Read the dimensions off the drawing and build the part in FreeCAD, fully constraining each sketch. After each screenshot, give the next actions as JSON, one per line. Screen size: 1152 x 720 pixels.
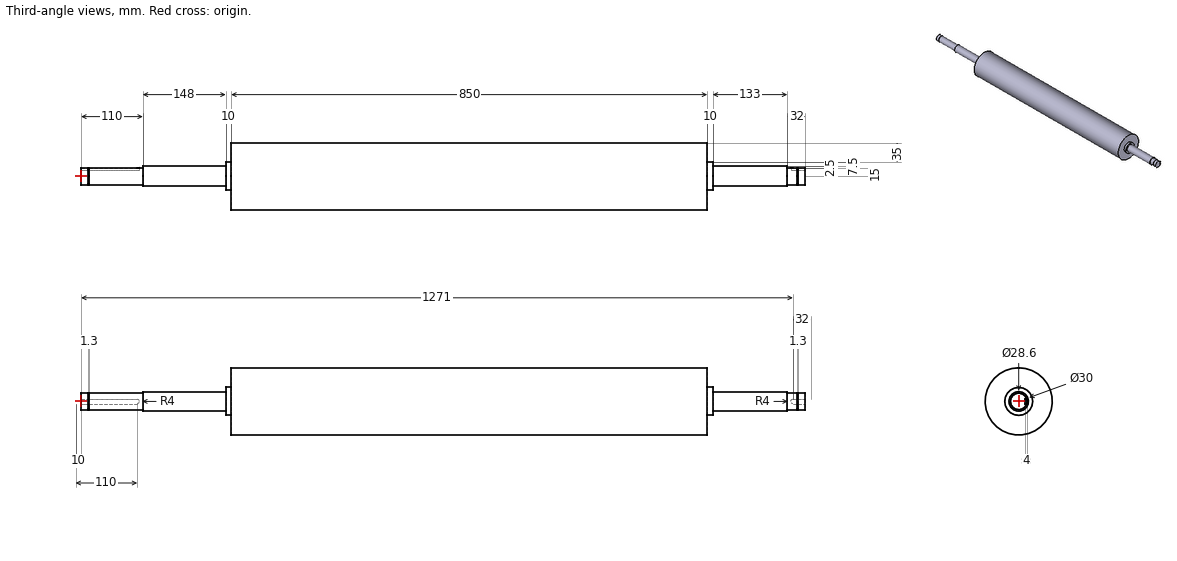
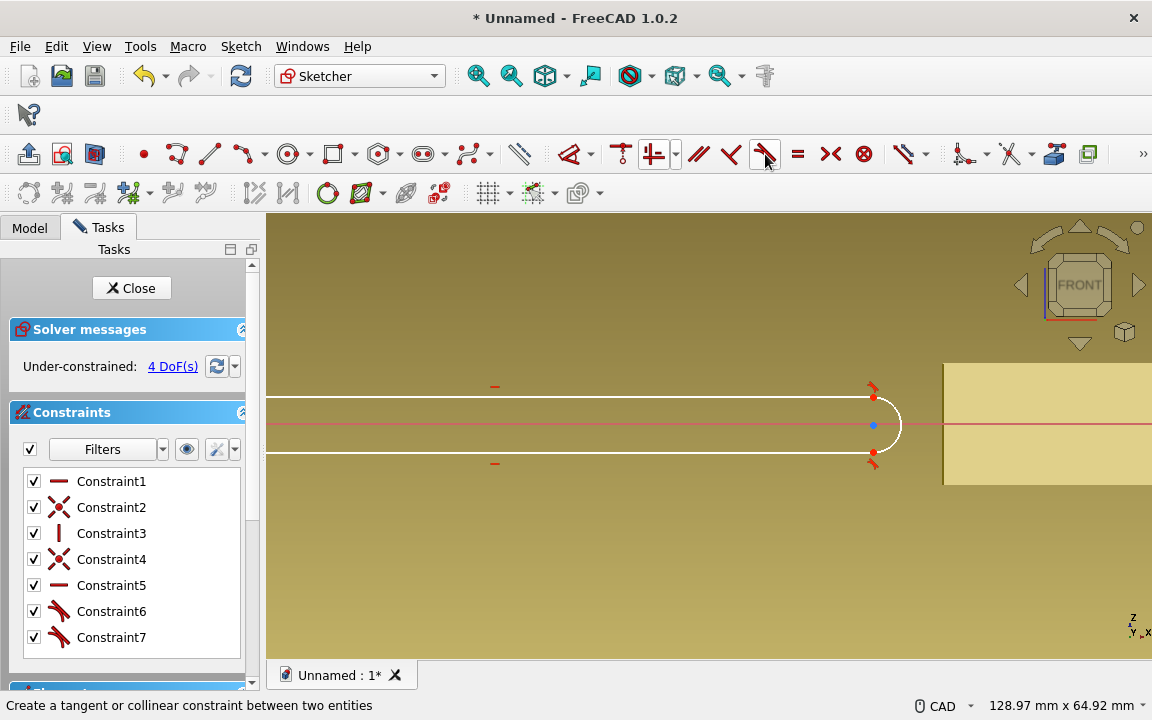
{"action": "left_click", "coordinate": [873, 425]}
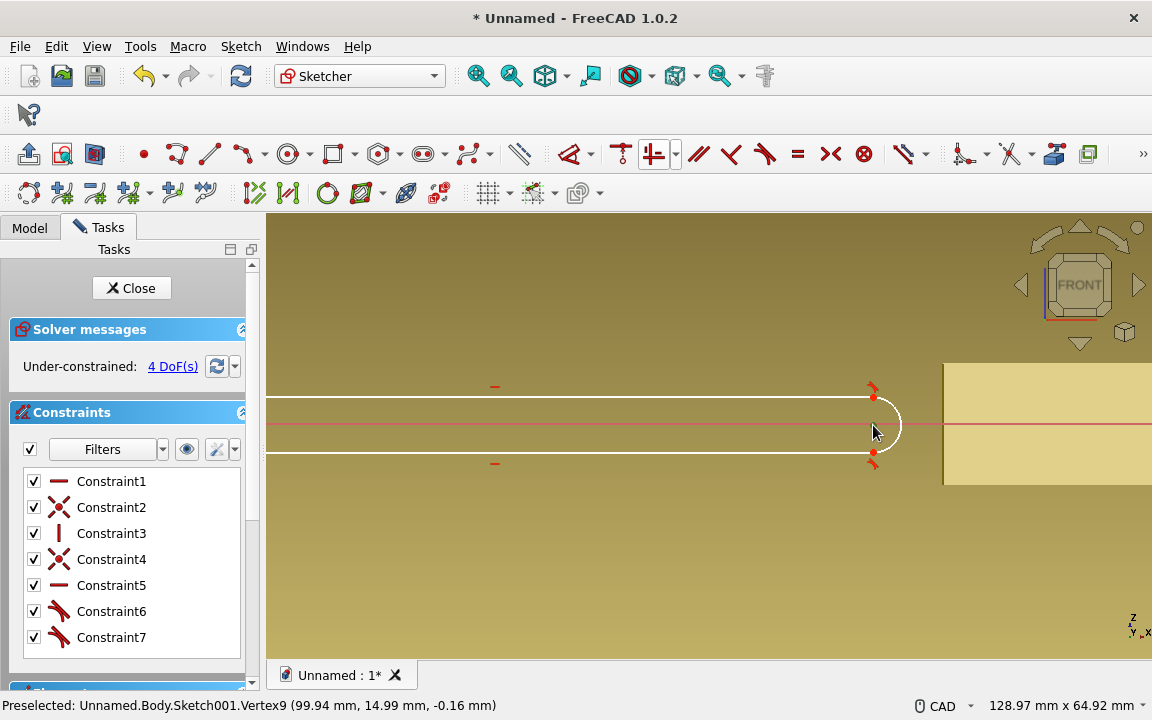
{"action": "left_click", "coordinate": [938, 424]}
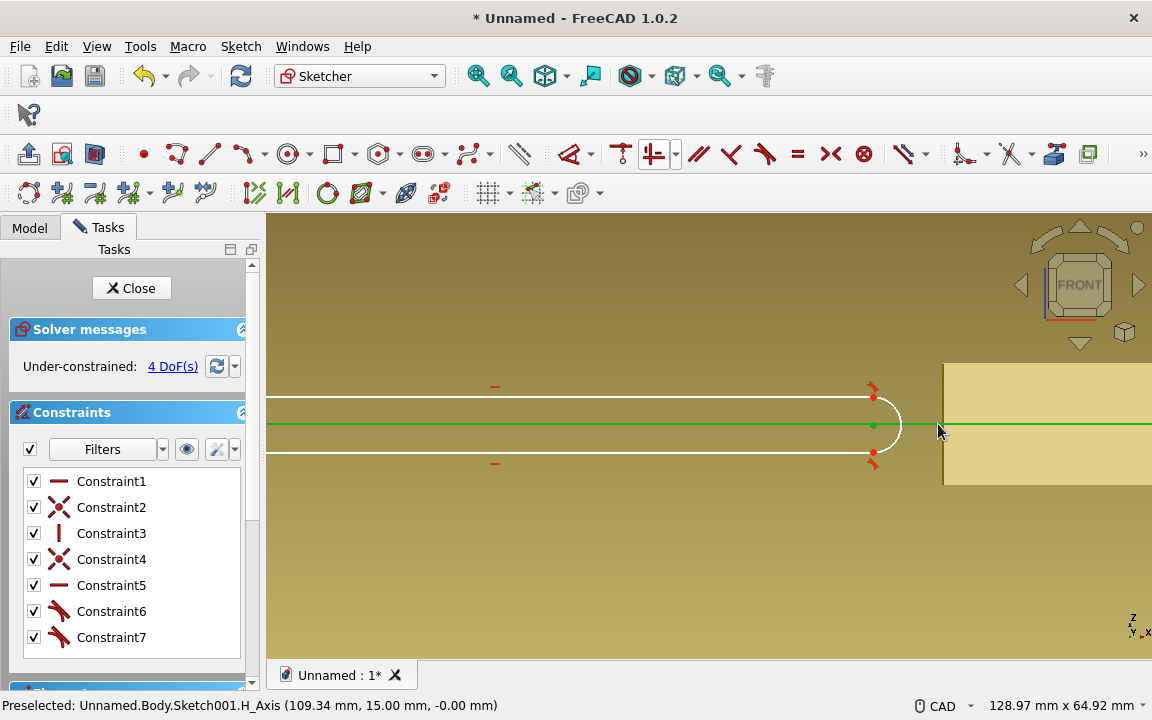
{"action": "left_click", "coordinate": [621, 154]}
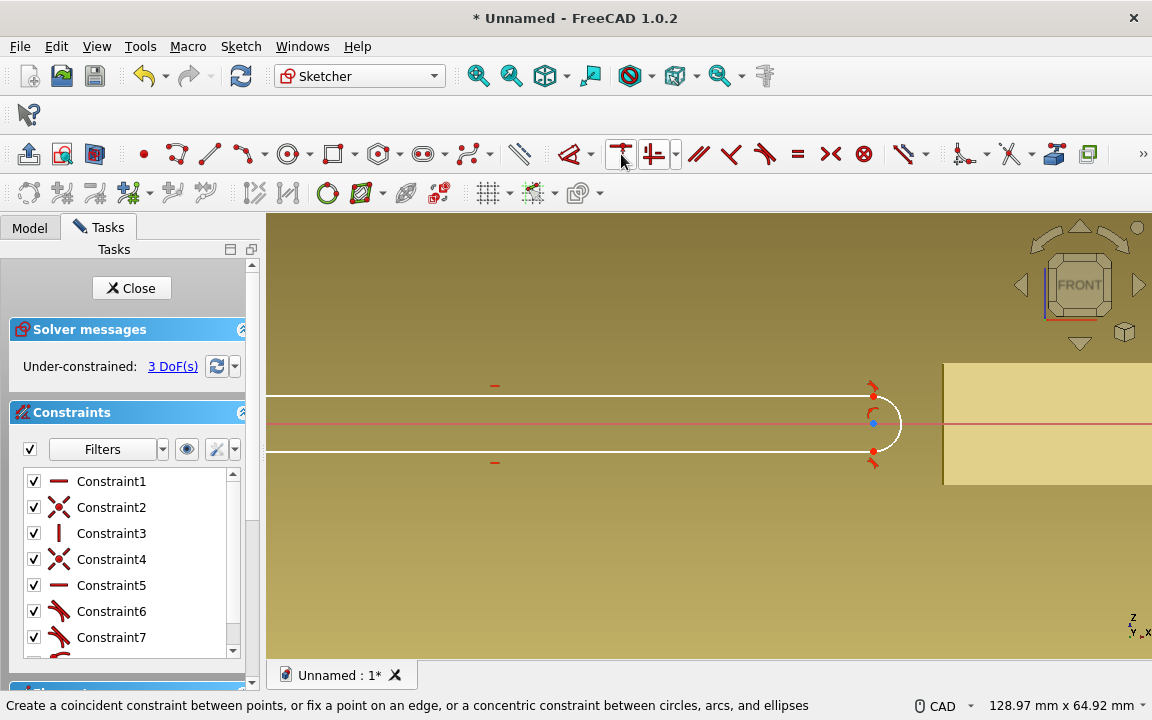
{"action": "key", "text": "d"}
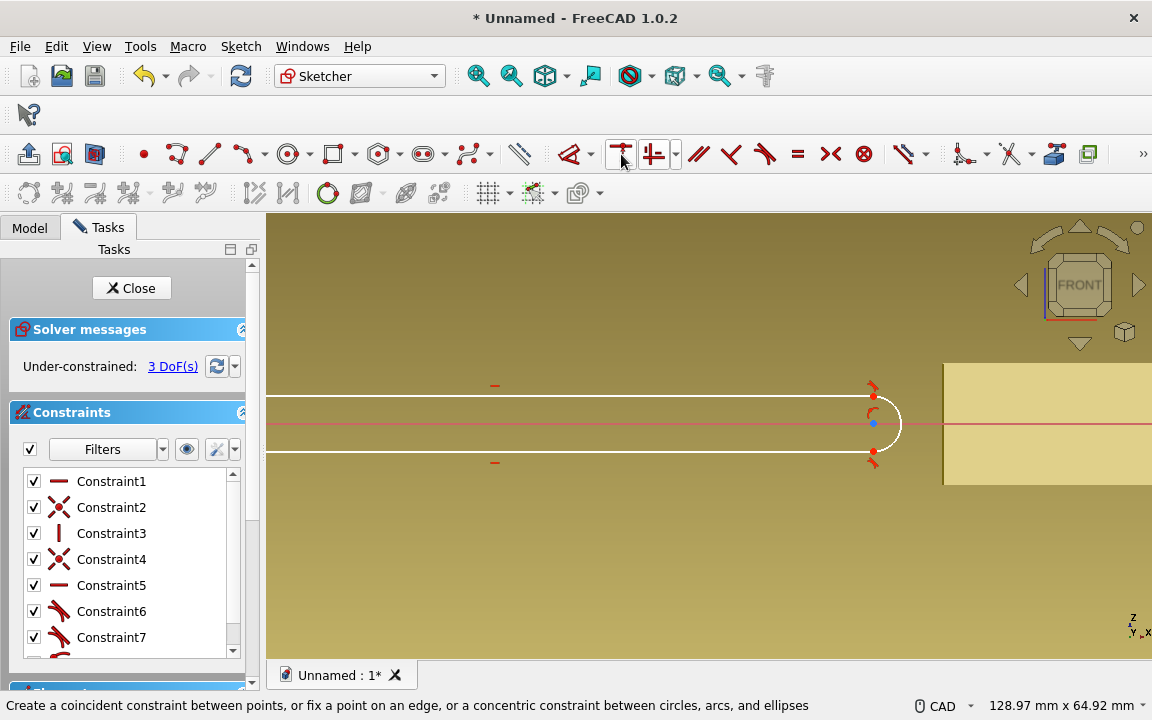
{"action": "scroll", "coordinate": [896, 440], "scroll_direction": "up", "scroll_amount": 2}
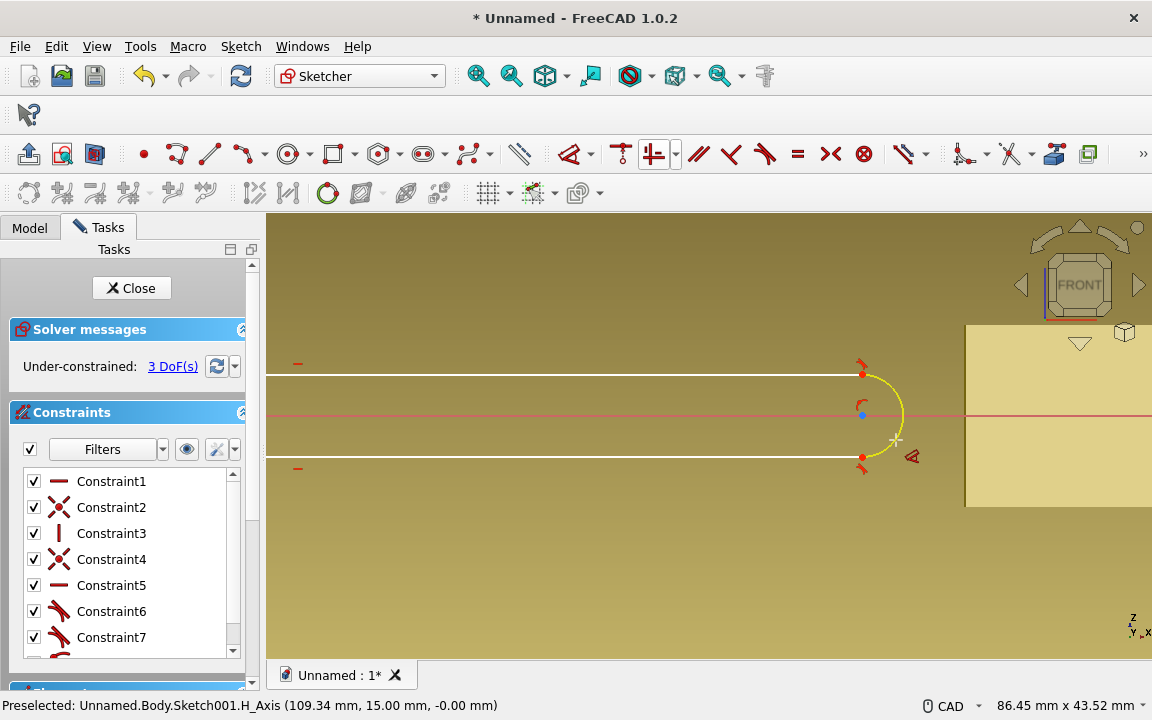
{"action": "left_click", "coordinate": [895, 440]}
{"action": "left_click", "coordinate": [921, 459]}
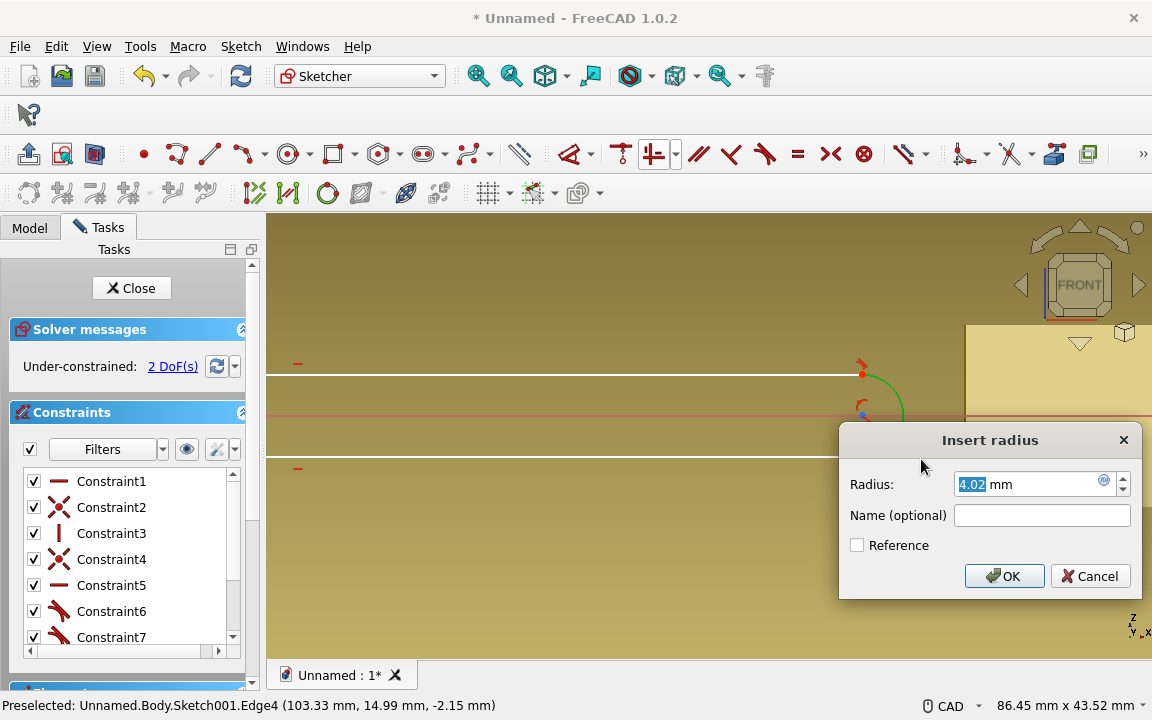
{"action": "type", "text": "4"}
{"action": "key", "text": "Return"}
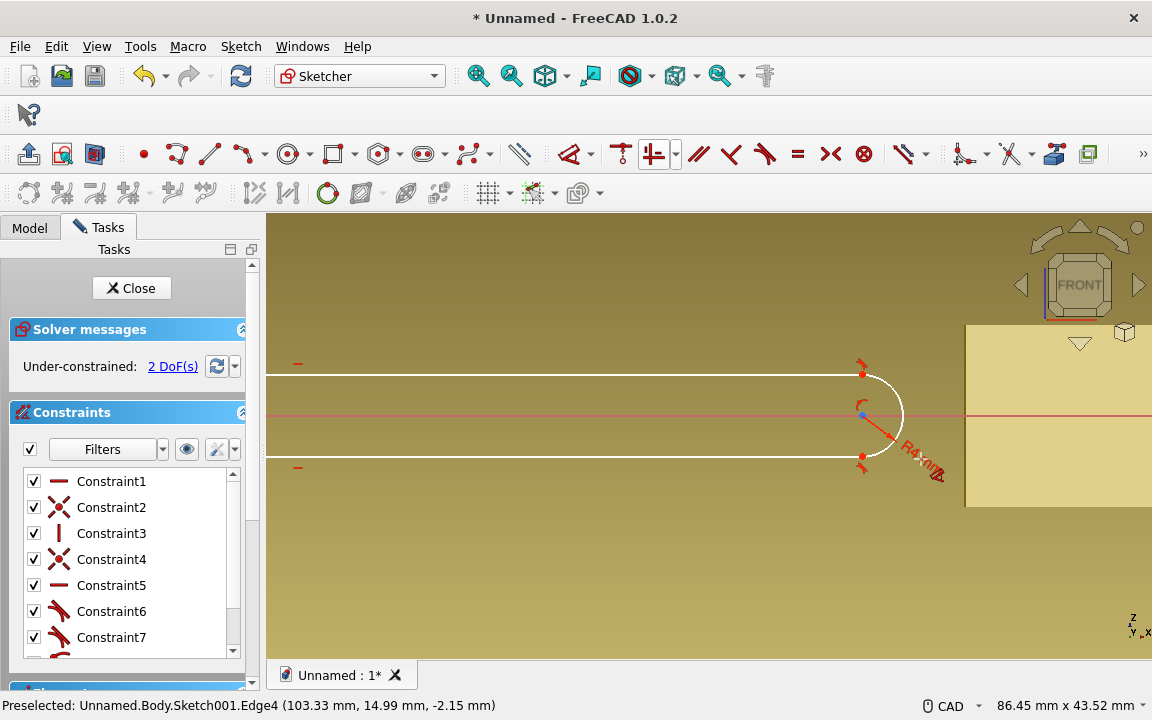
{"action": "left_click", "coordinate": [524, 457]}
{"action": "left_click", "coordinate": [578, 491]}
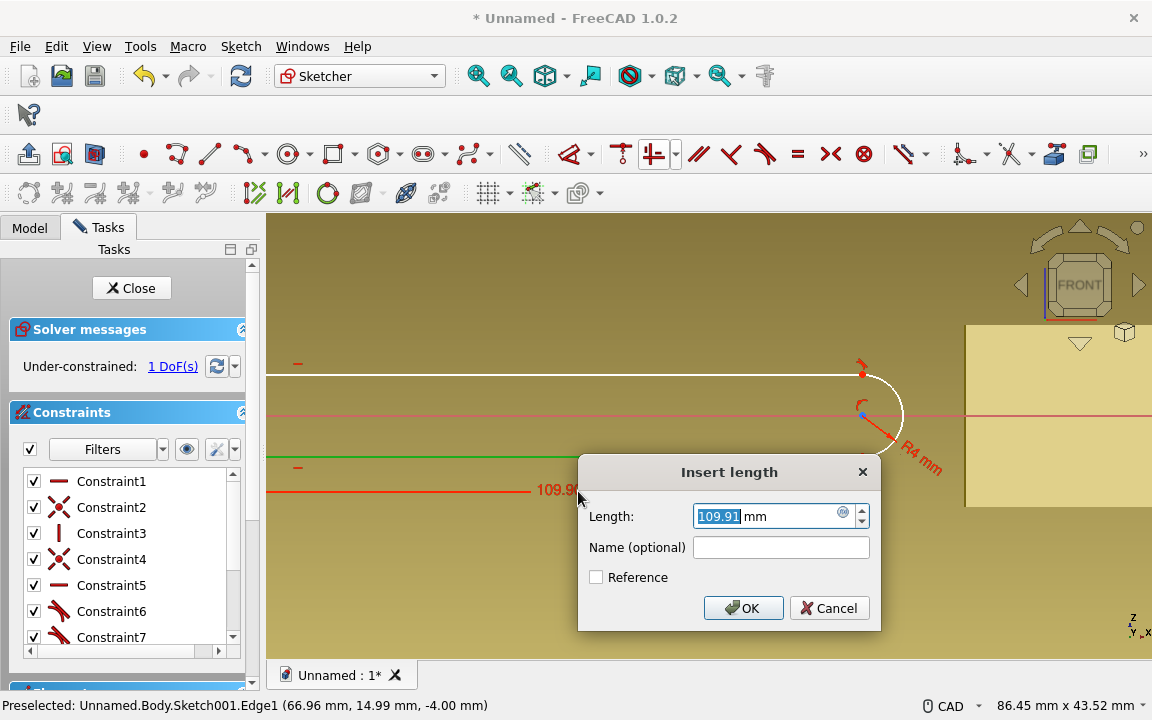
{"action": "type", "text": "110"}
{"action": "key", "text": "Return"}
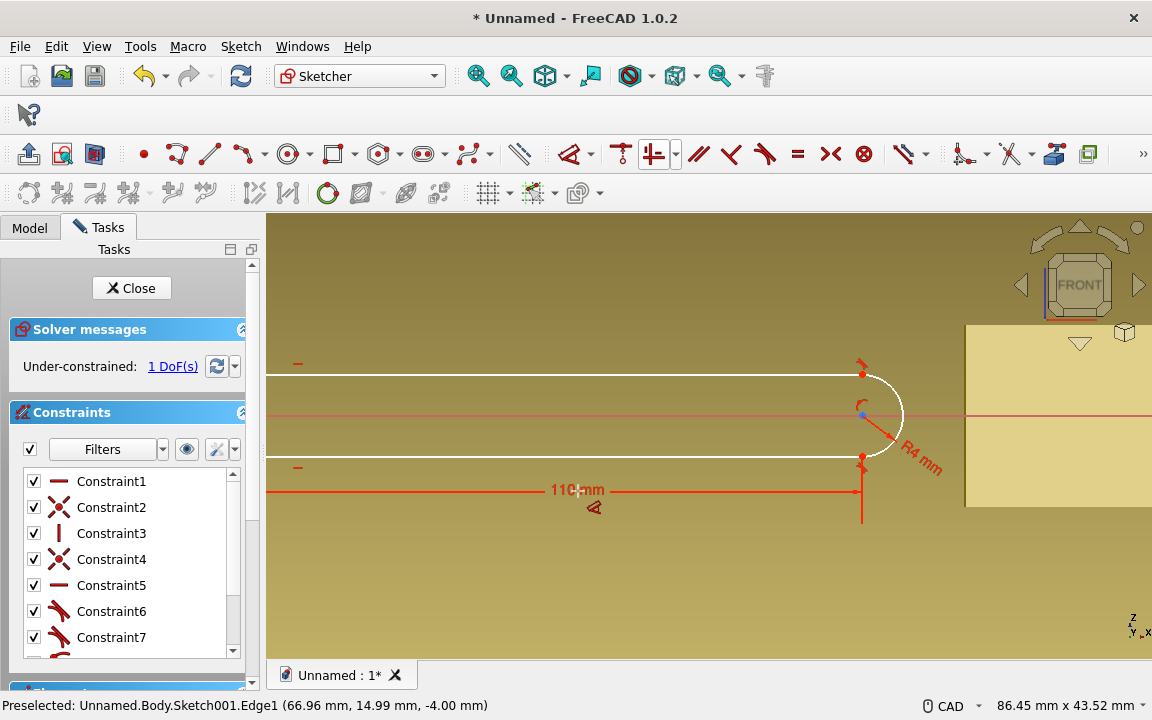
{"action": "scroll", "coordinate": [902, 452], "scroll_direction": "down", "scroll_amount": 4}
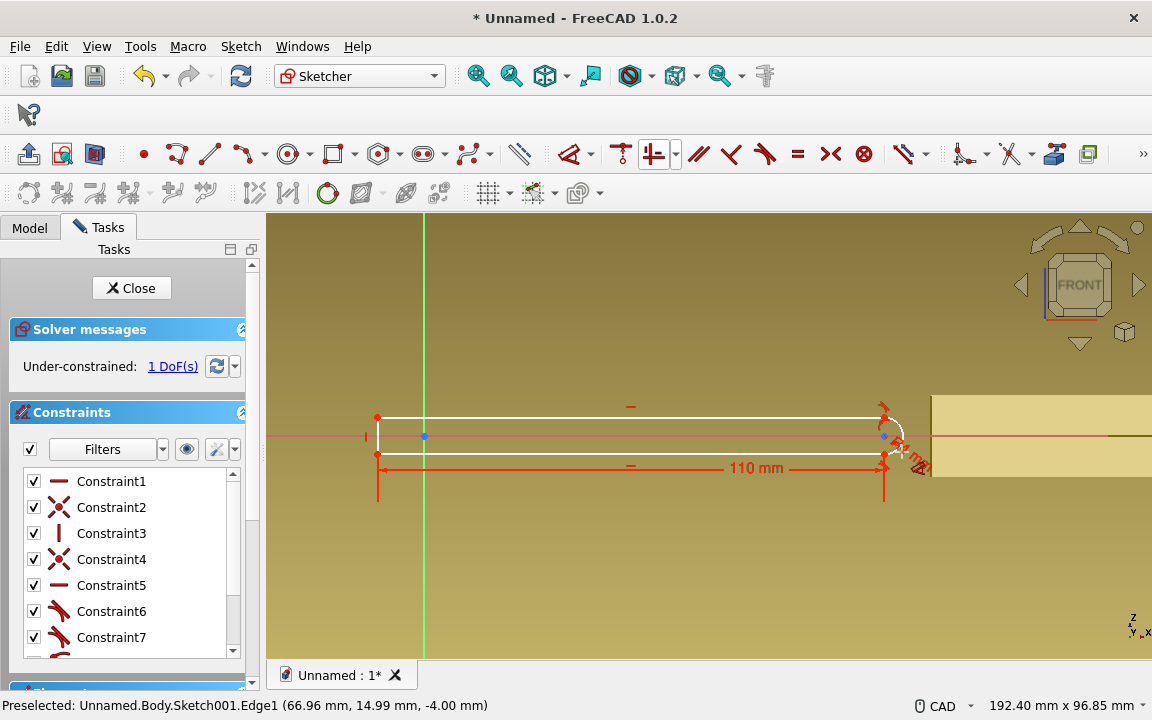
{"action": "left_click", "coordinate": [378, 454]}
{"action": "left_click", "coordinate": [401, 488]}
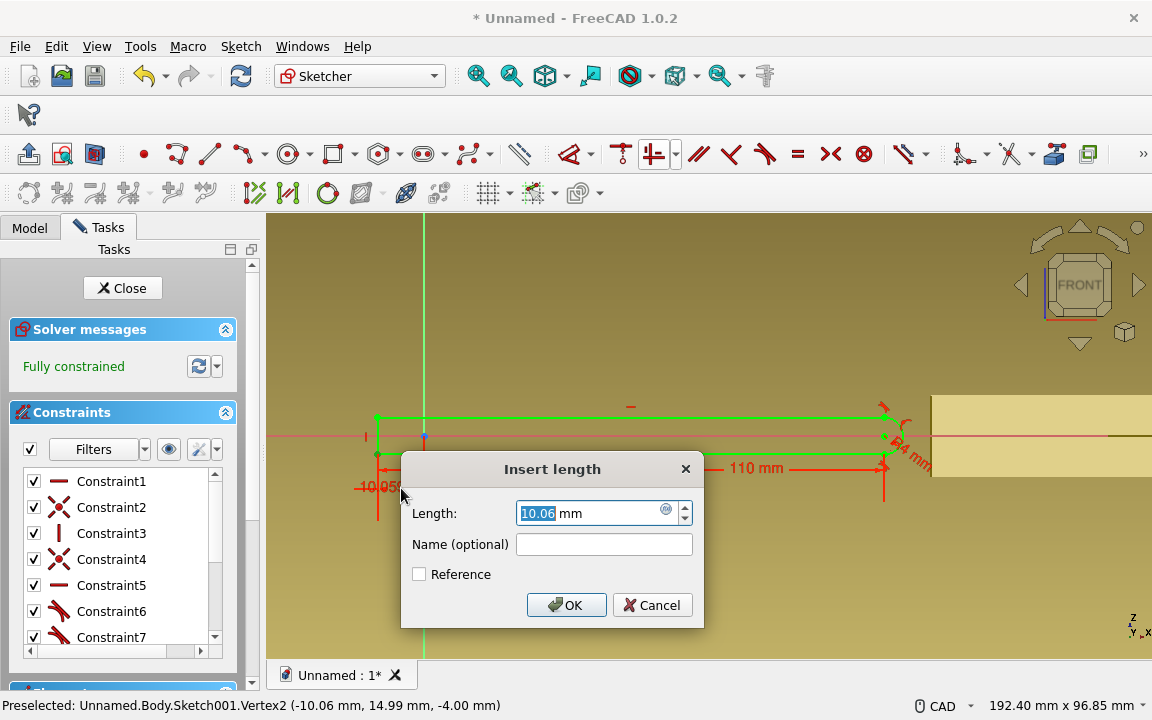
{"action": "type", "text": "10"}
{"action": "key", "text": "Return"}
{"action": "key", "text": "Escape"}